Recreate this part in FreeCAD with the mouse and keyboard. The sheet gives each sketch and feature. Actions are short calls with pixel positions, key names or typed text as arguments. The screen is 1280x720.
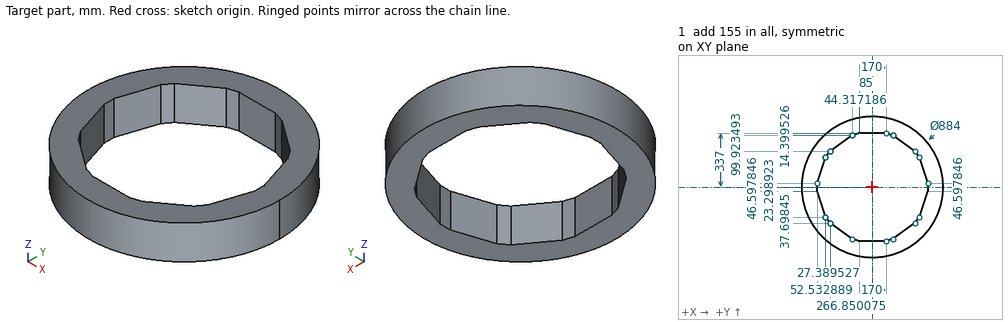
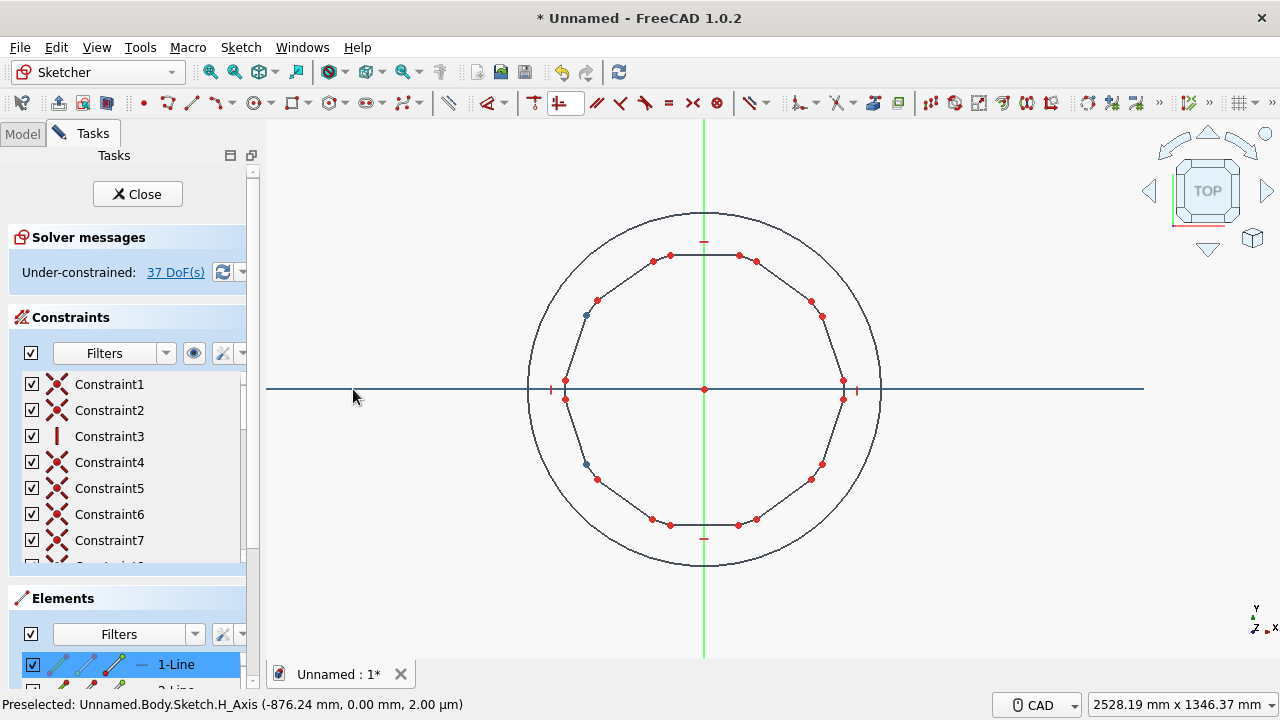
key(s)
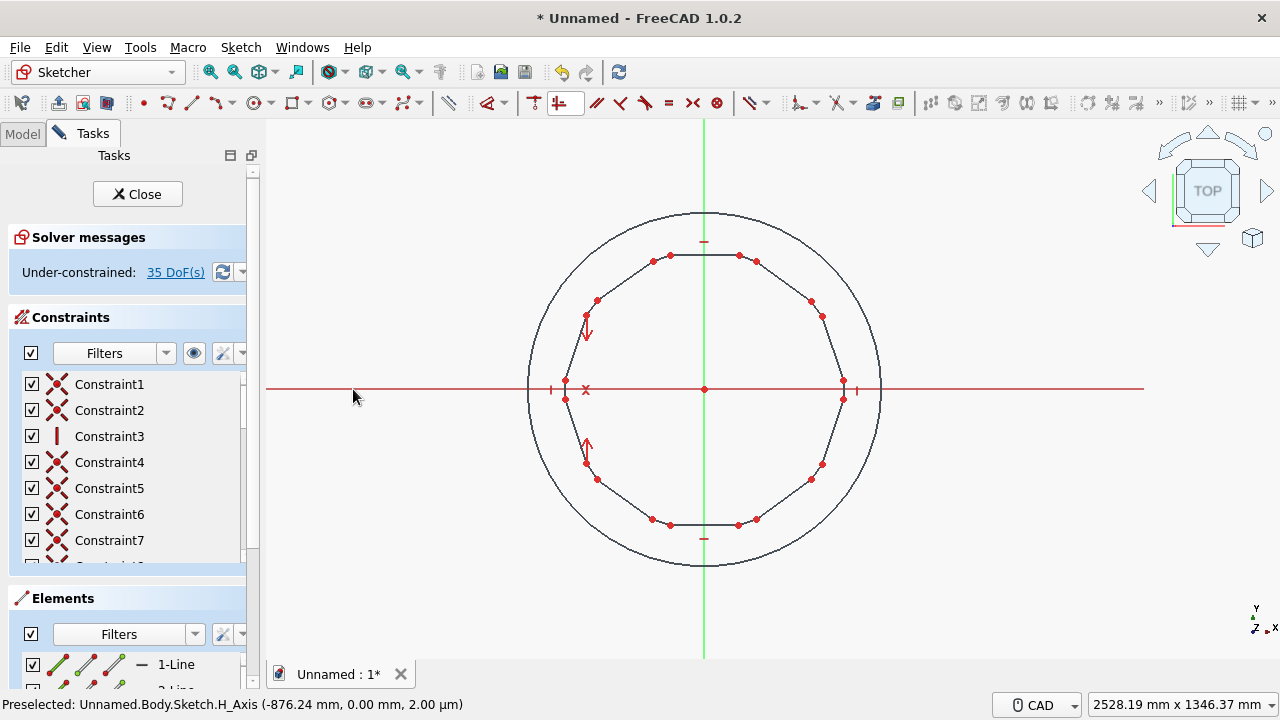
click(598, 480)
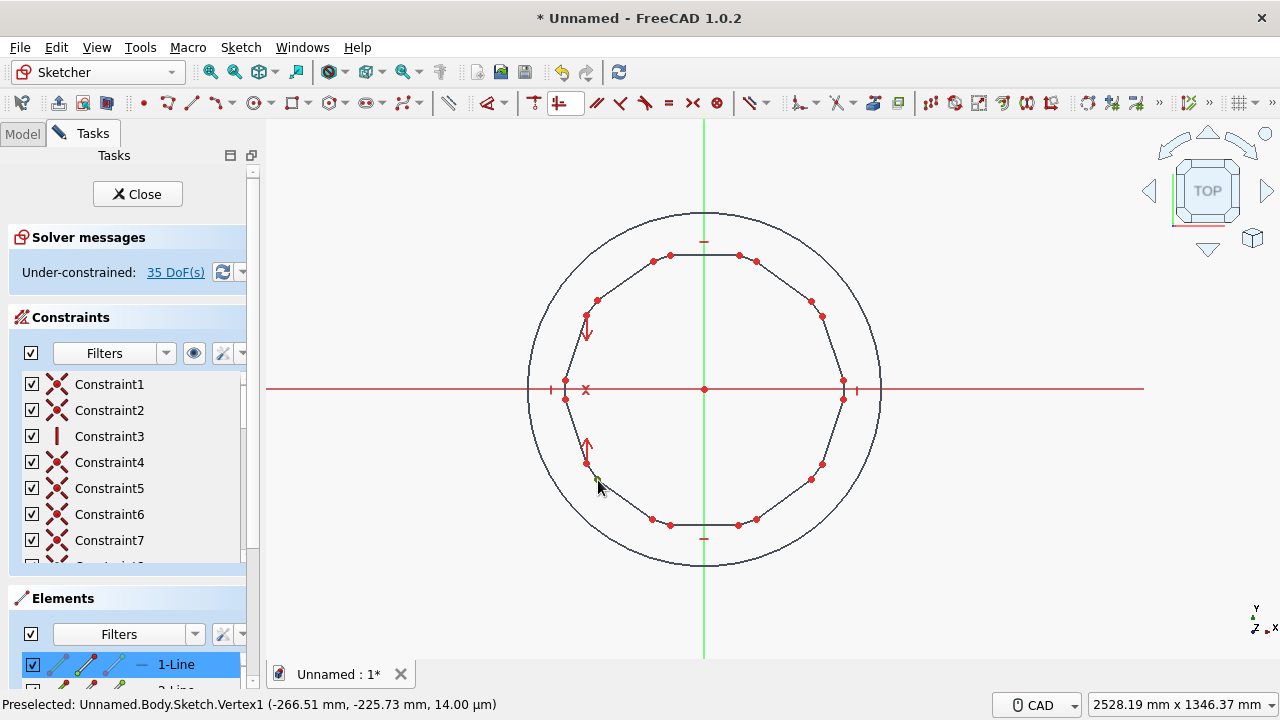
click(598, 300)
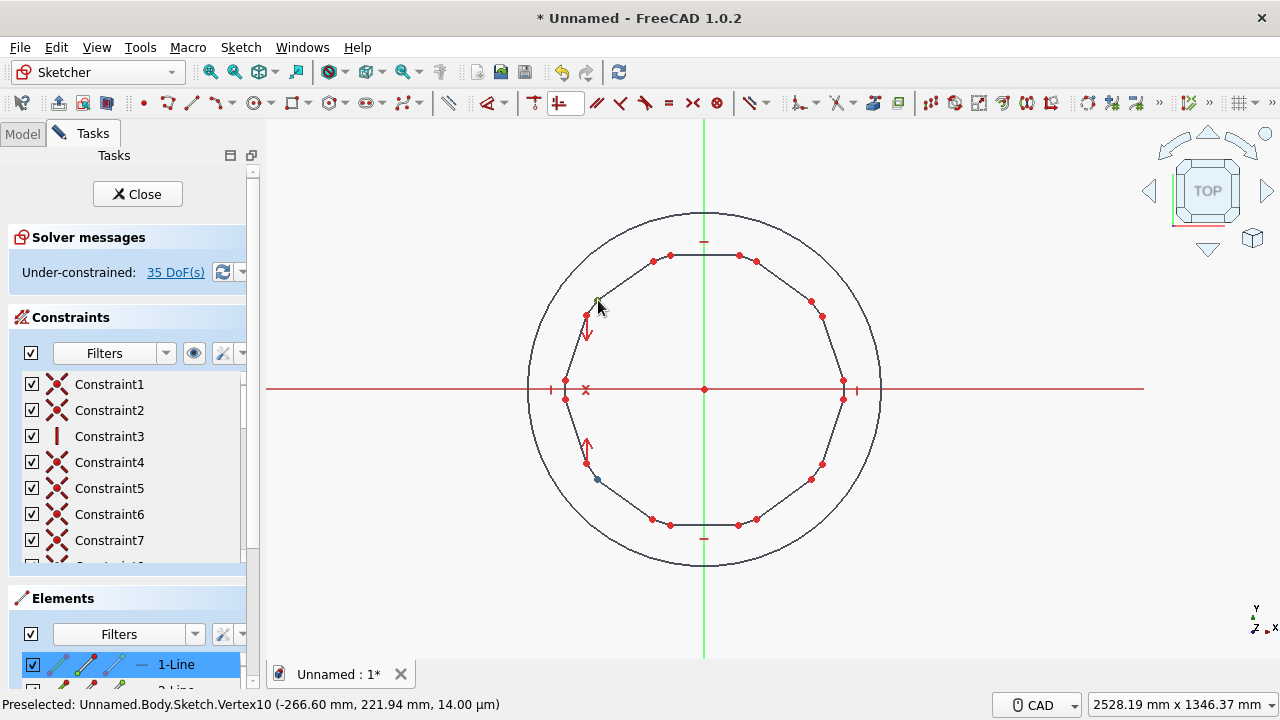
click(353, 389)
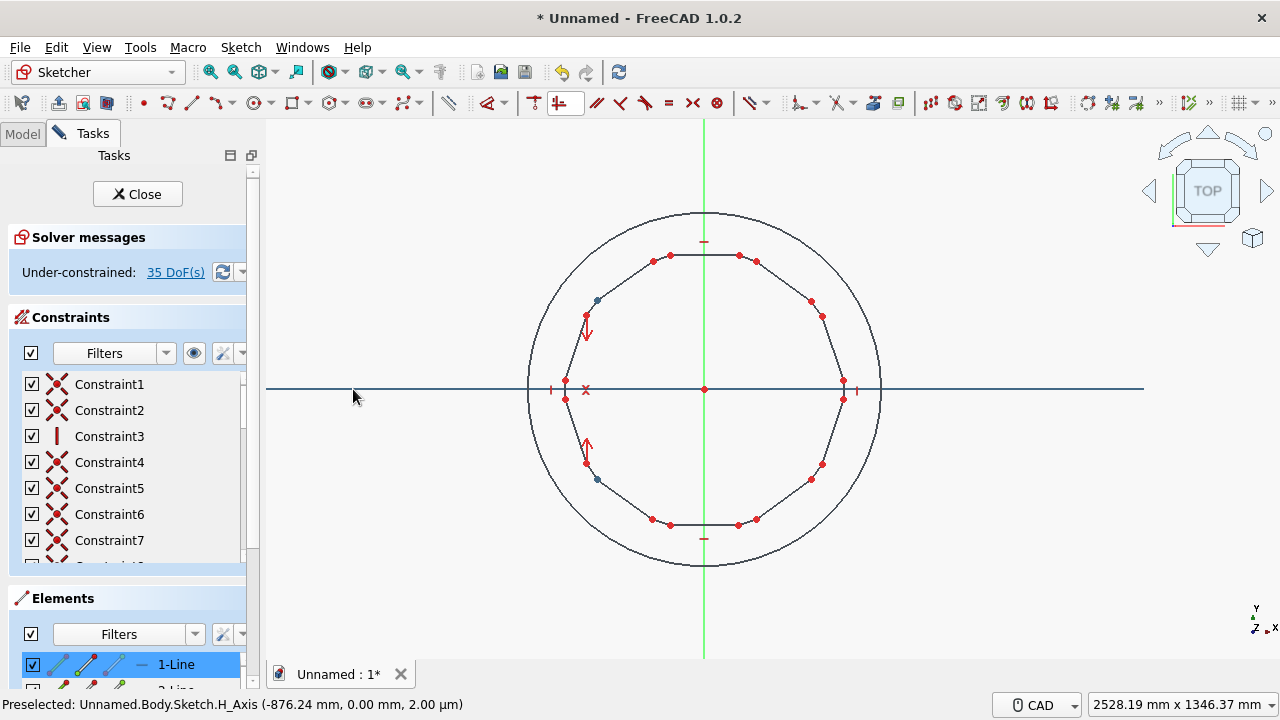
key(s)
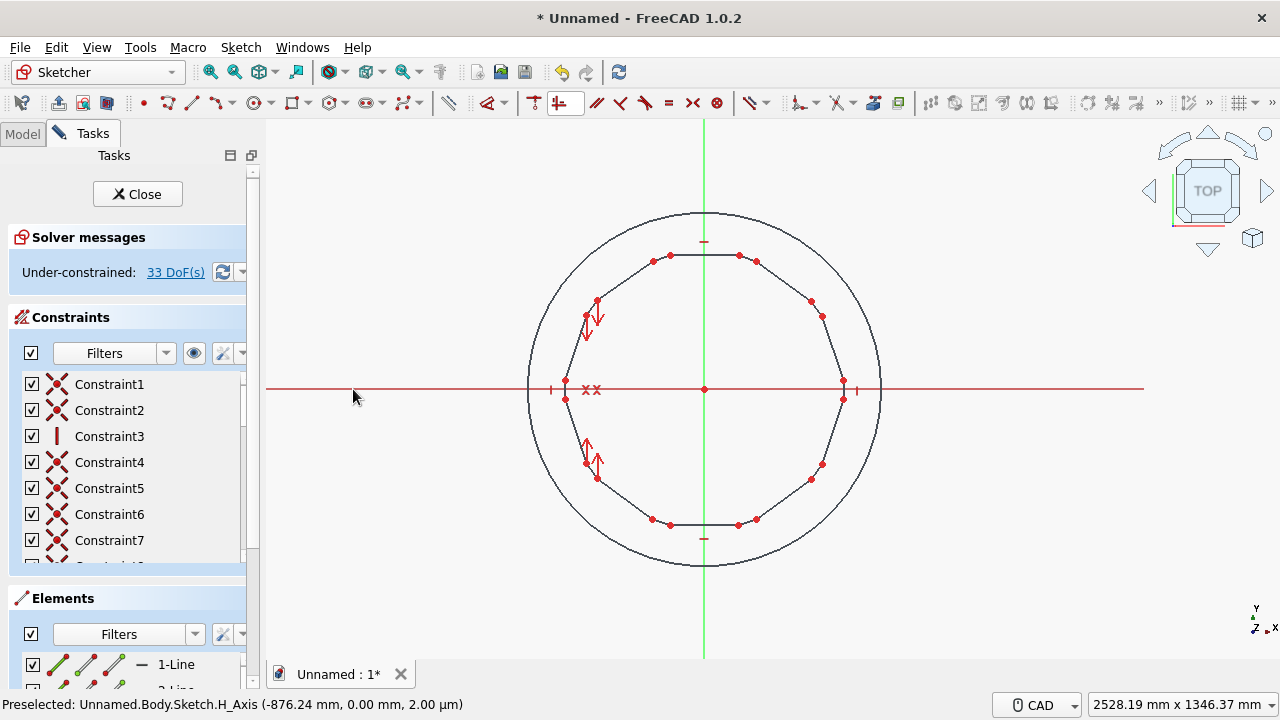
click(653, 261)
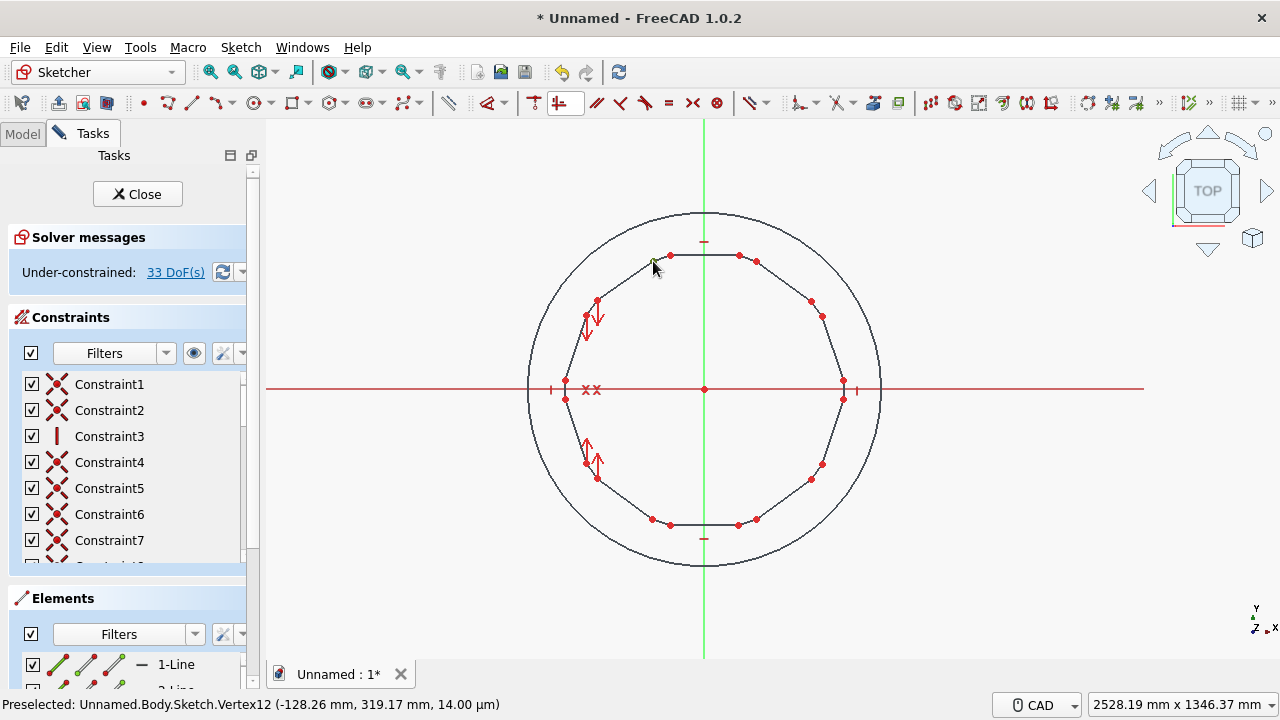
click(756, 261)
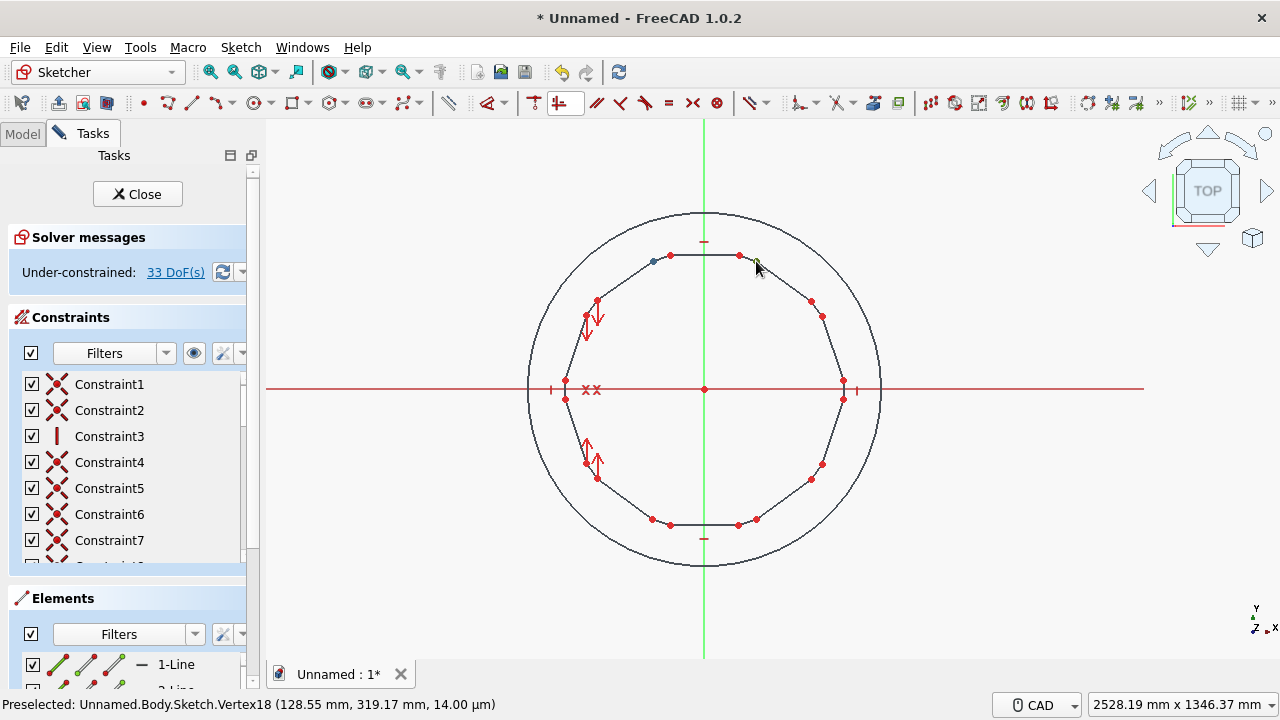
click(704, 596)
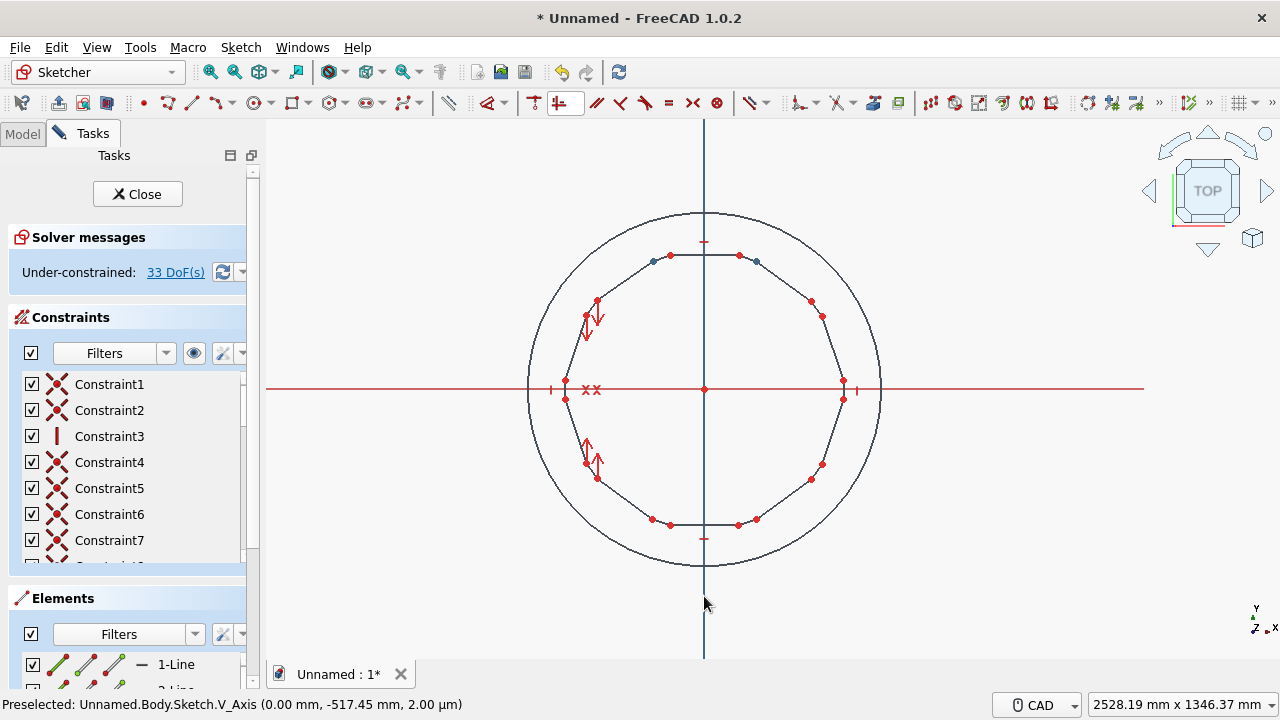
click(694, 104)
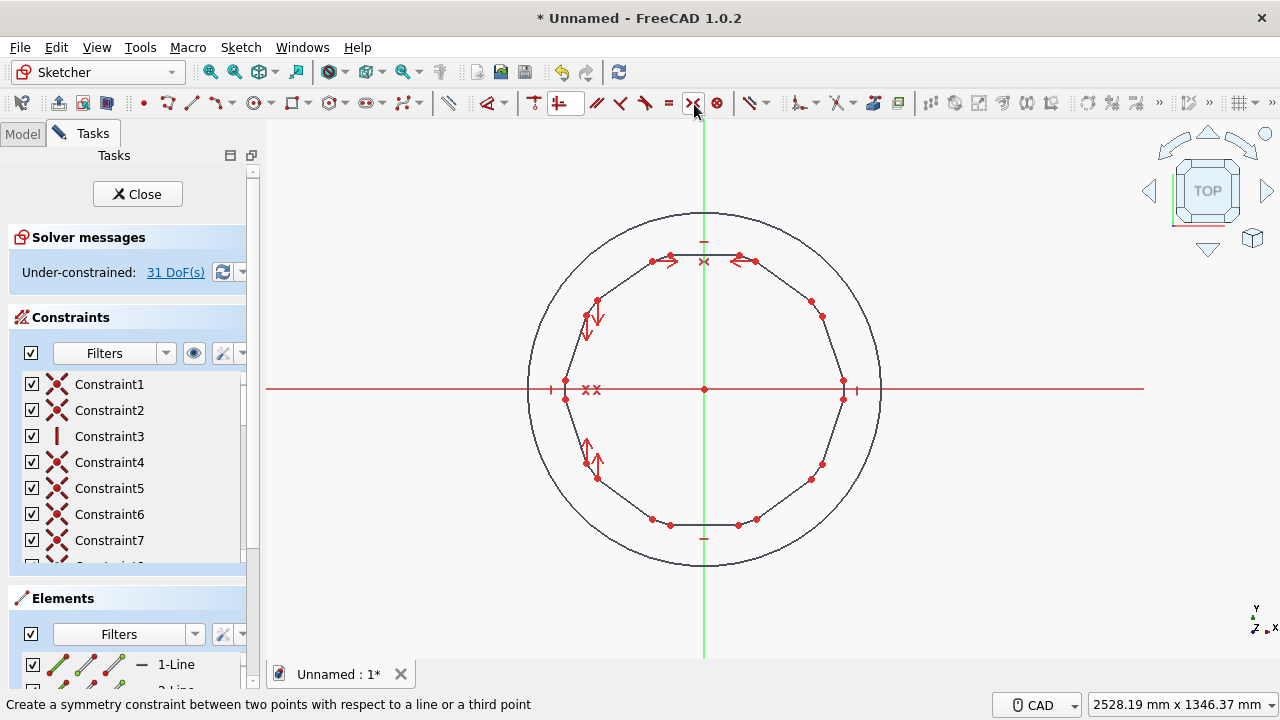
click(598, 300)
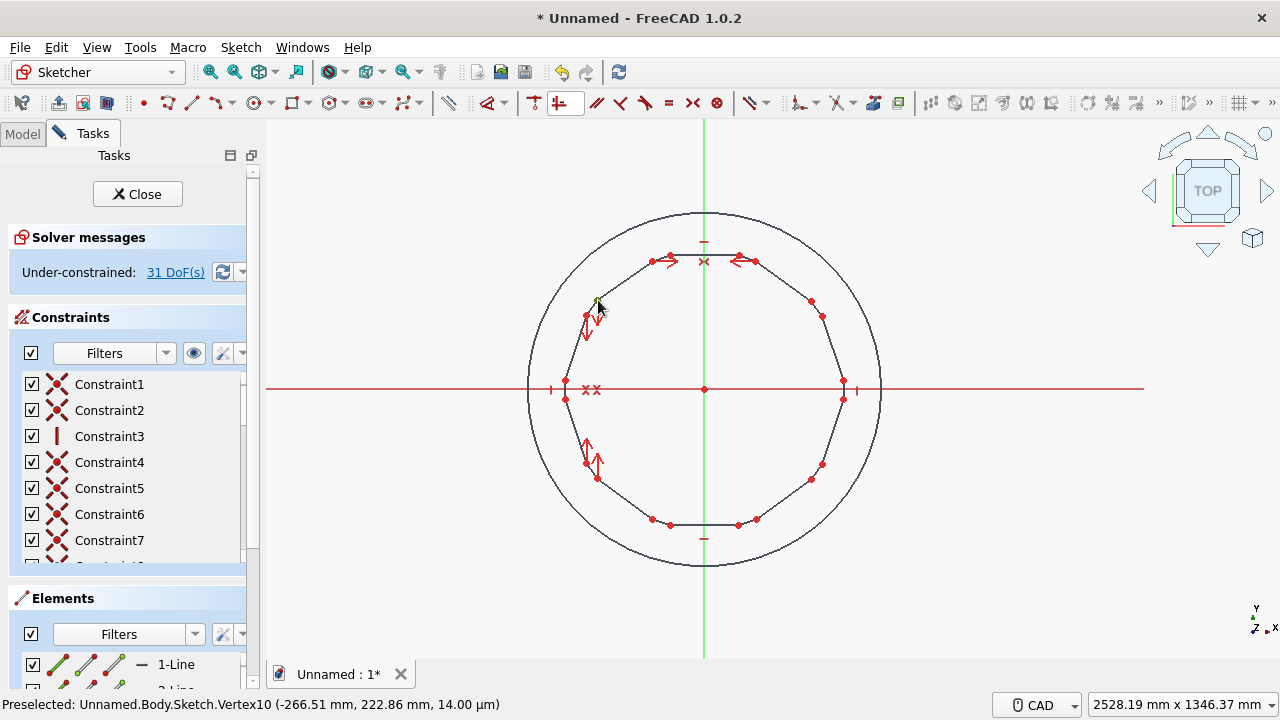
click(811, 301)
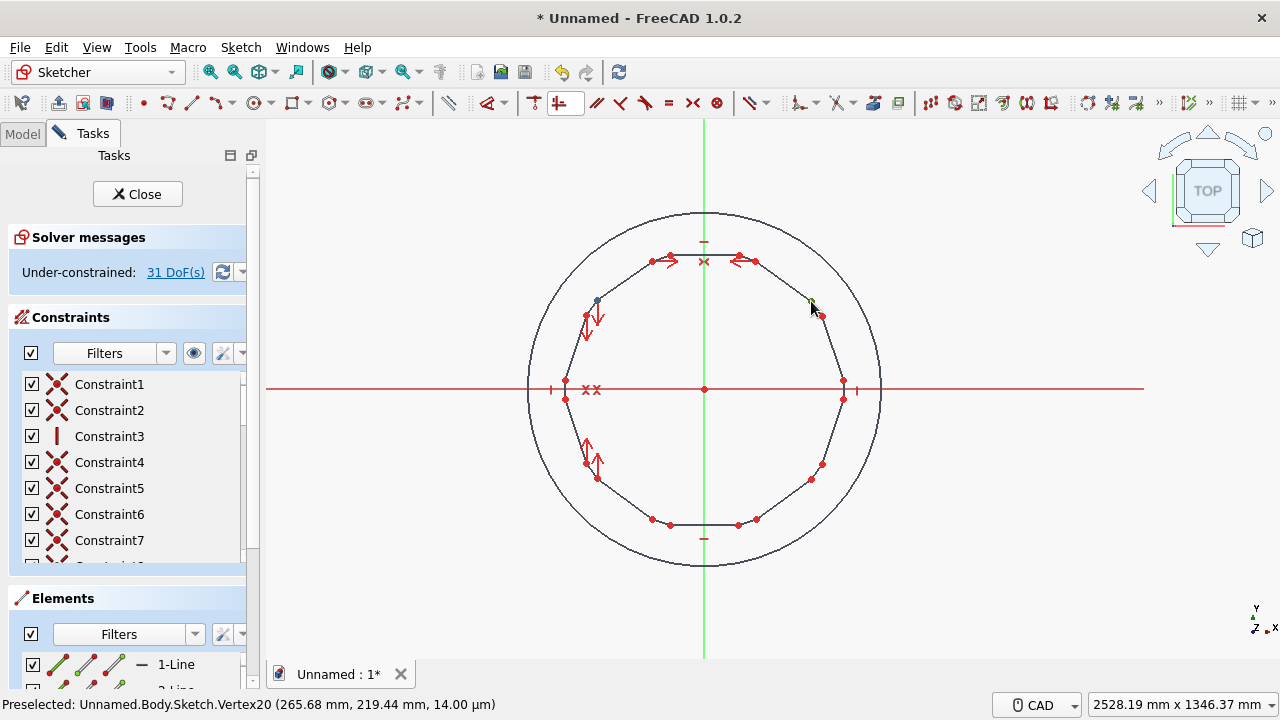
click(704, 596)